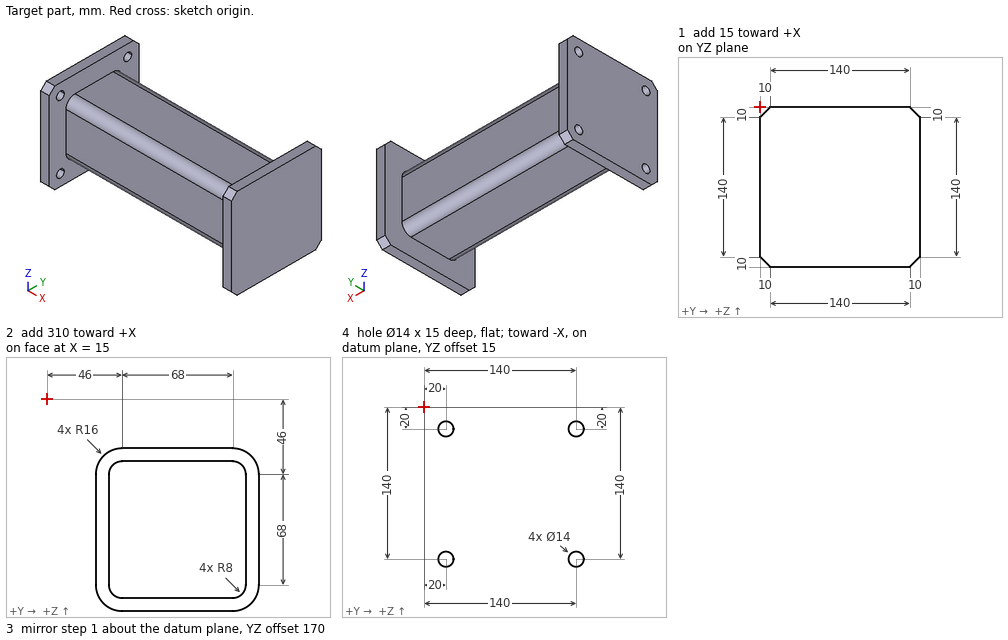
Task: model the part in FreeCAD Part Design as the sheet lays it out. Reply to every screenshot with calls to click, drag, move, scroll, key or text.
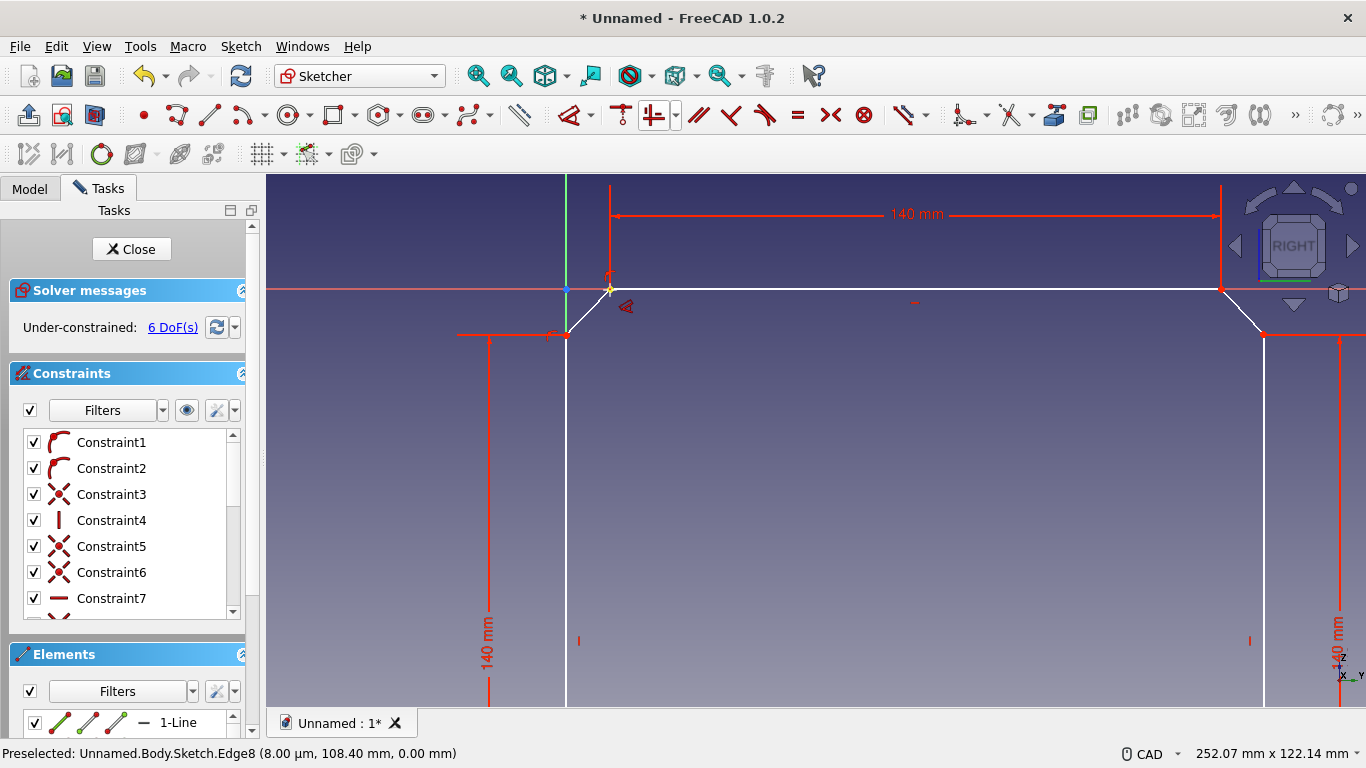
click(610, 289)
click(588, 255)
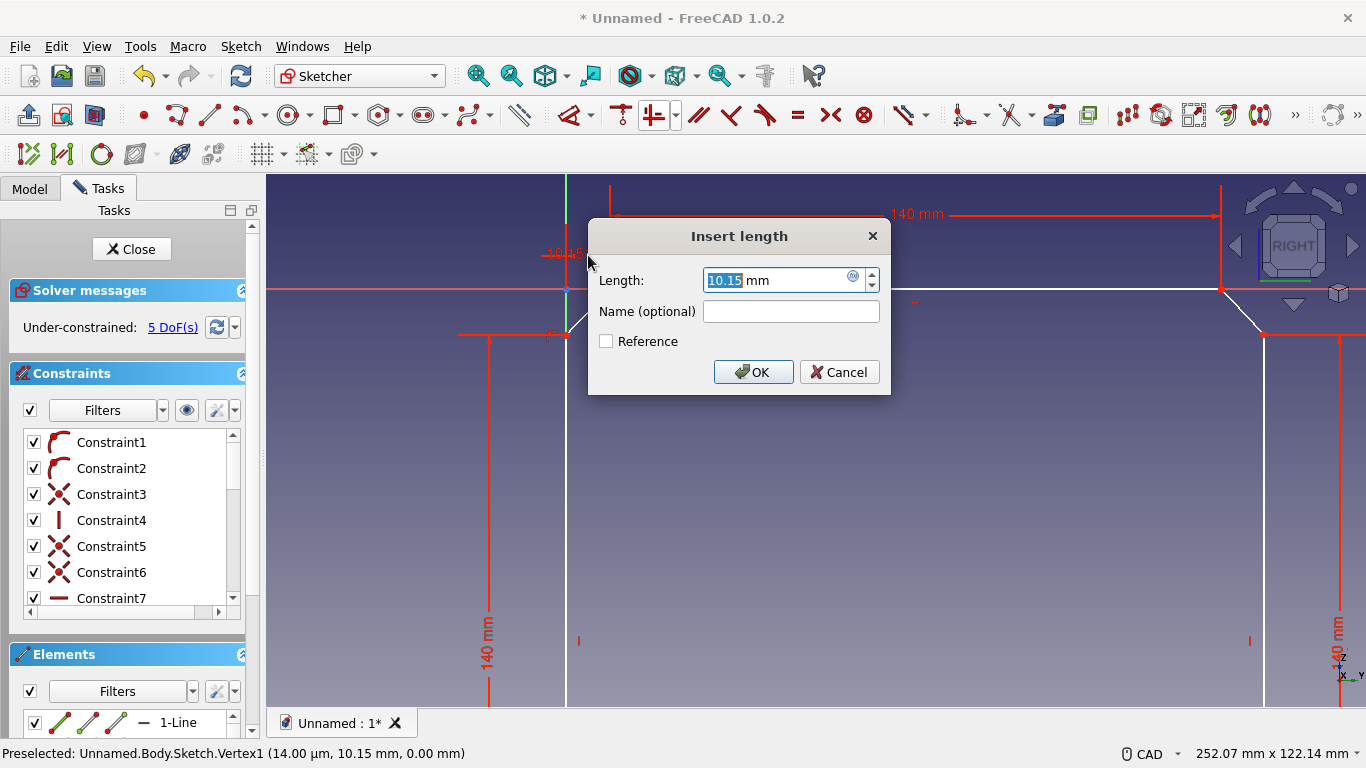
text(10)
key(Return)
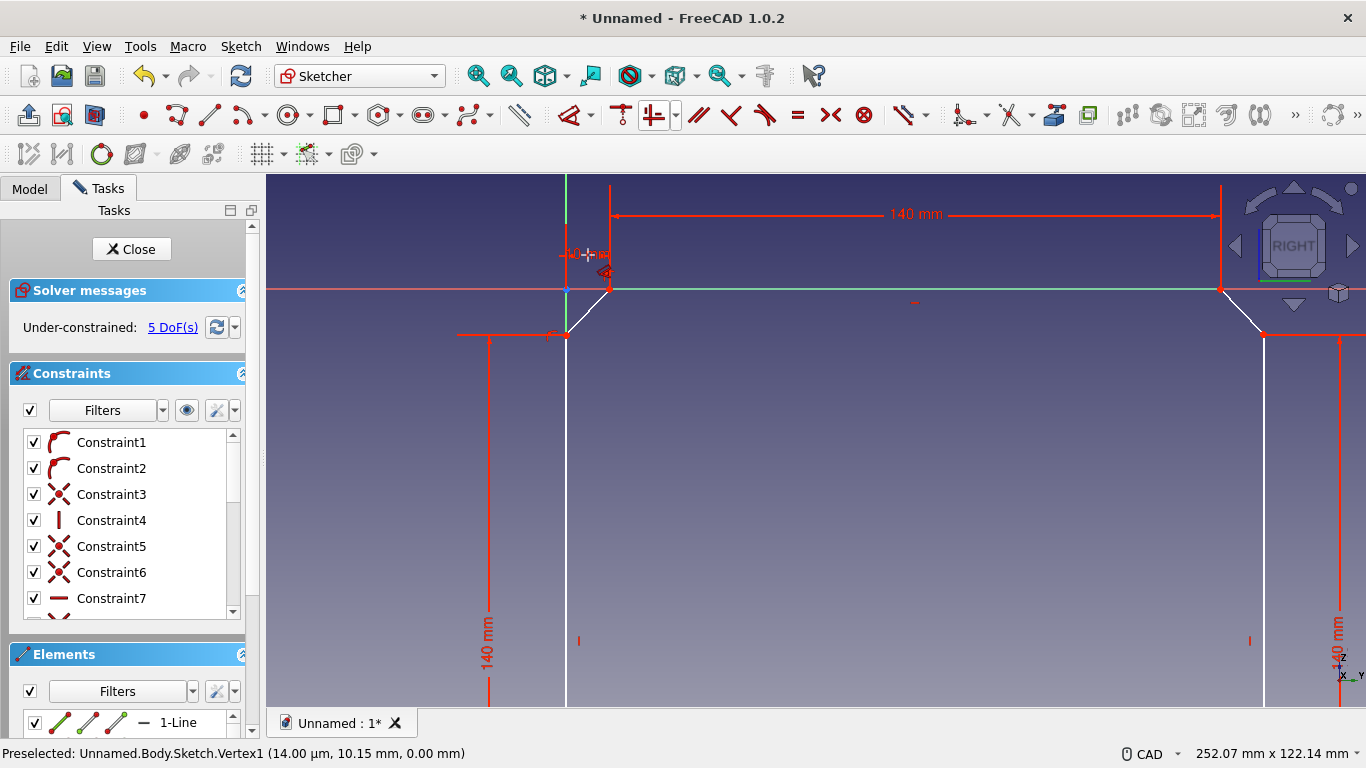
click(566, 335)
click(532, 312)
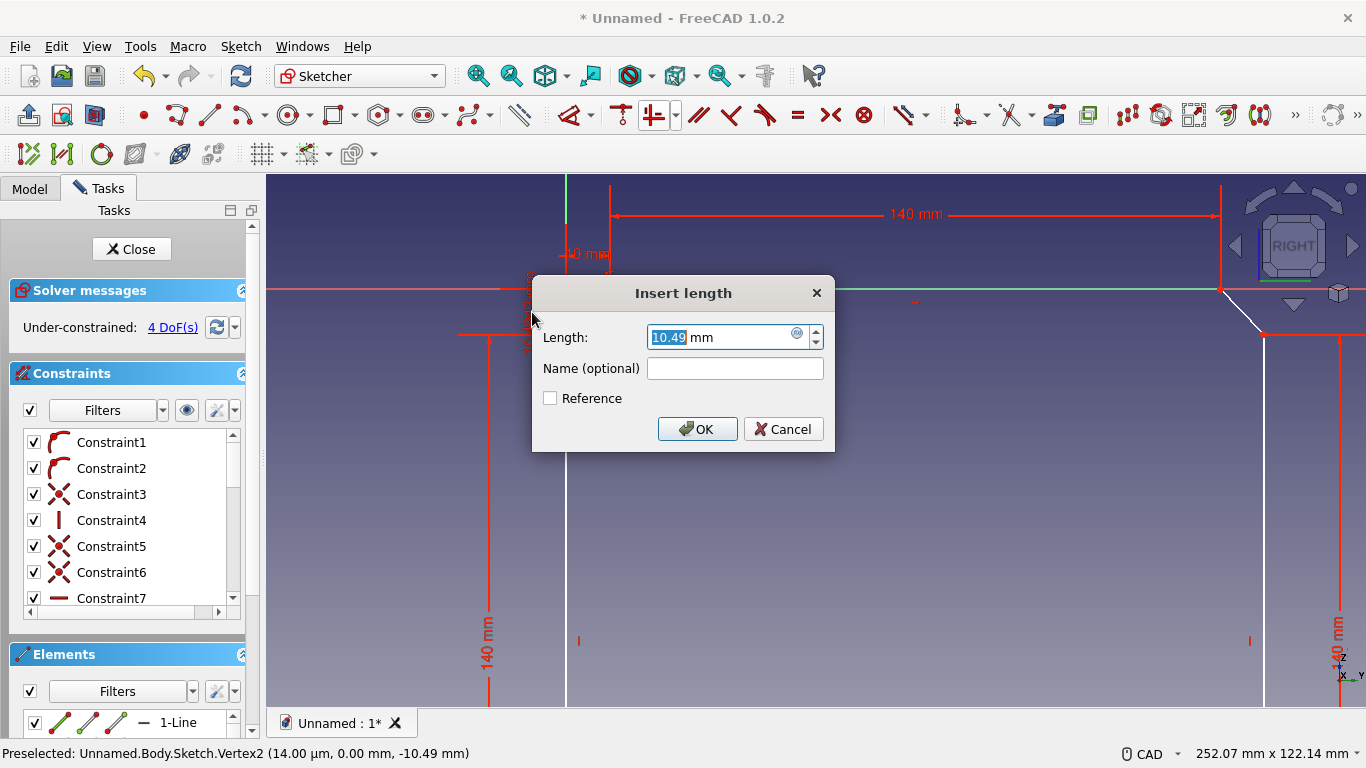
text(10)
key(Return)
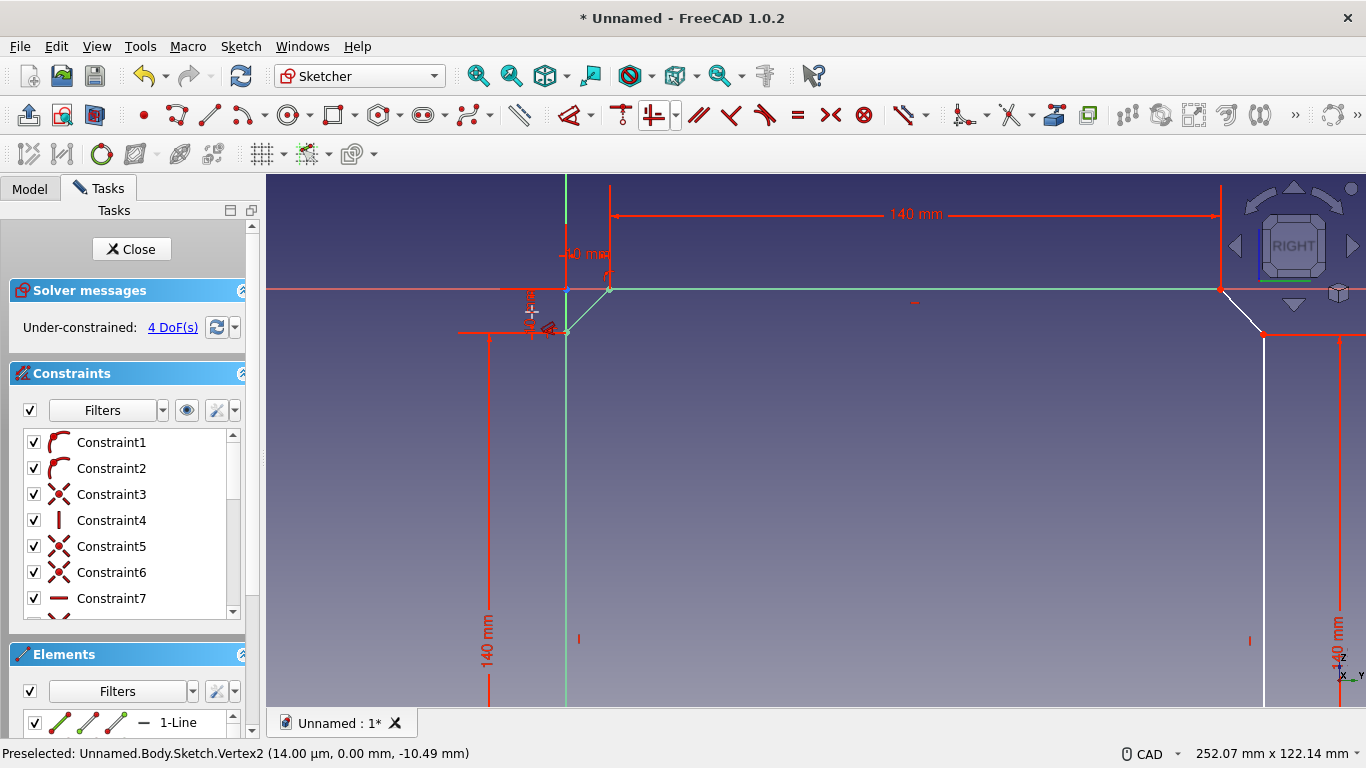
scroll(611, 279, down, 4)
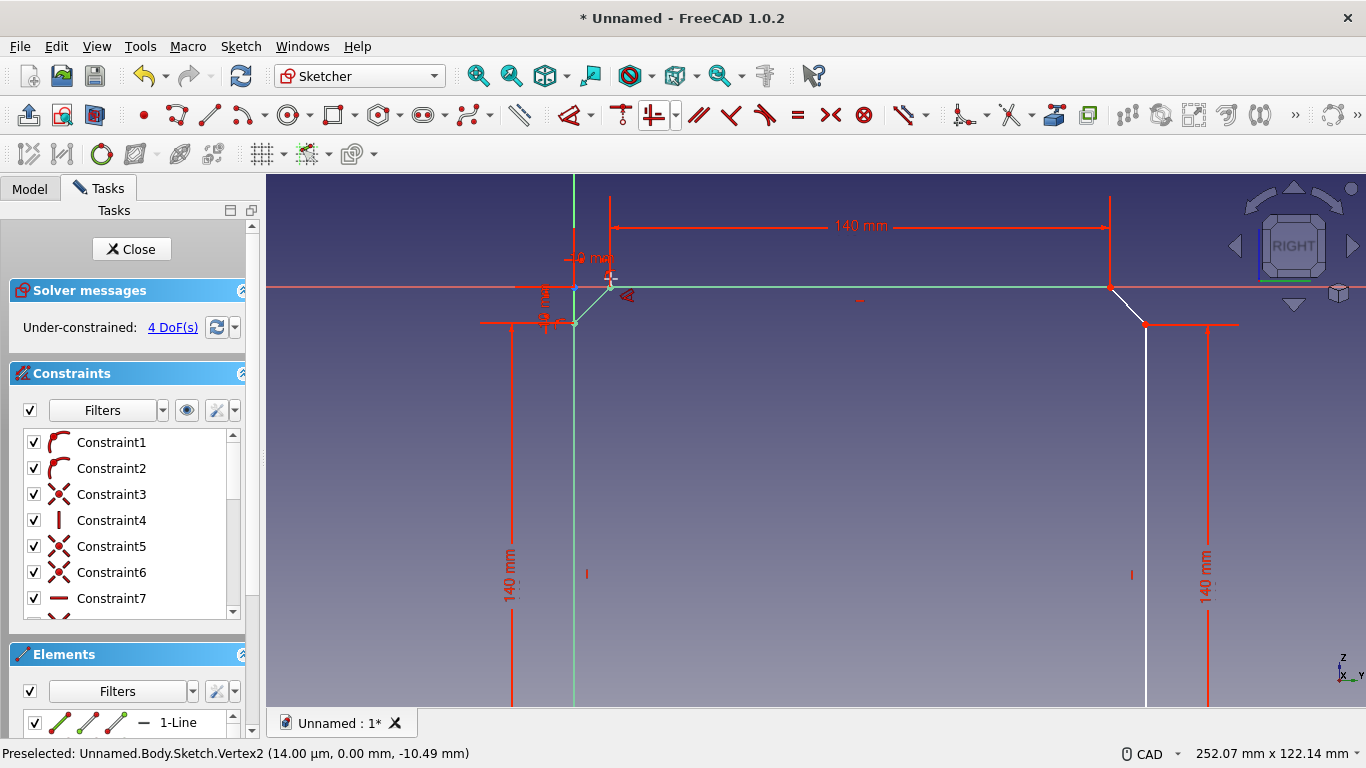
scroll(611, 599, up, 4)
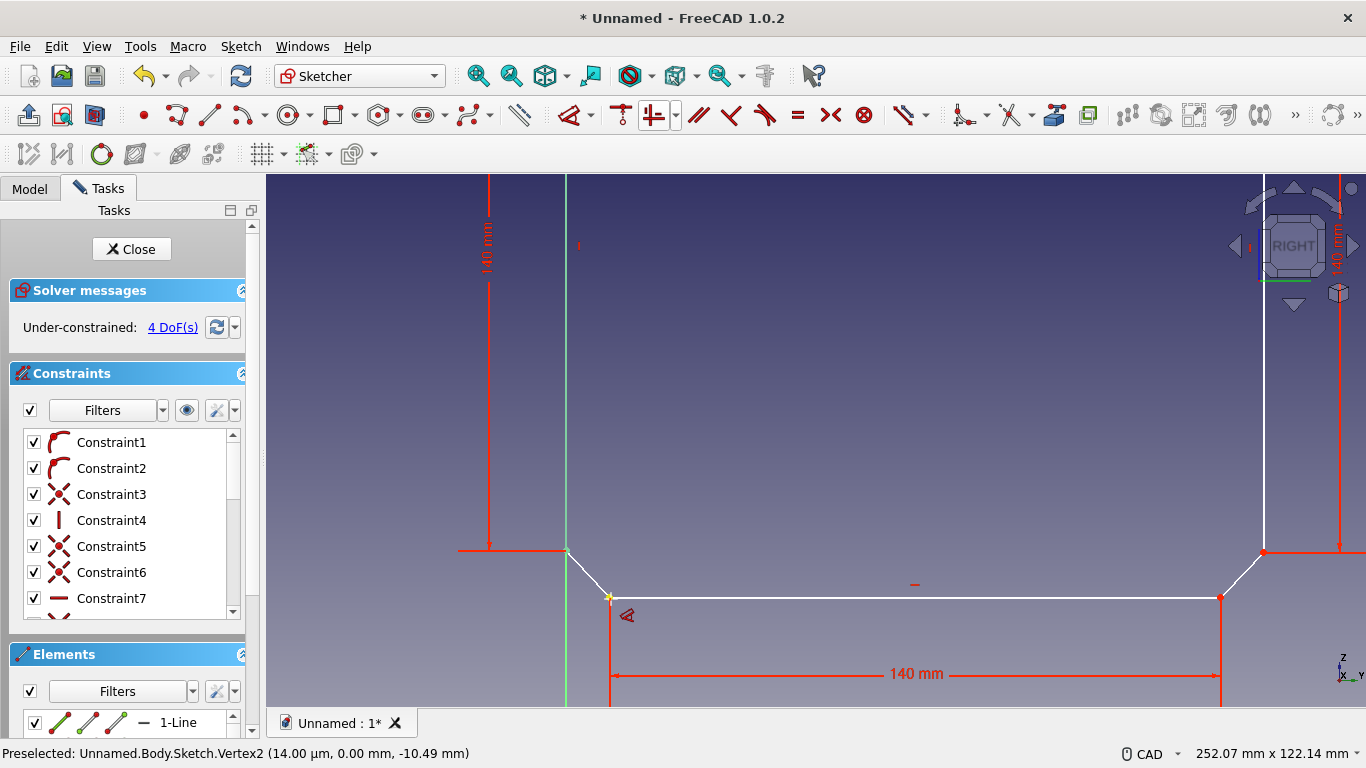
click(610, 598)
click(588, 632)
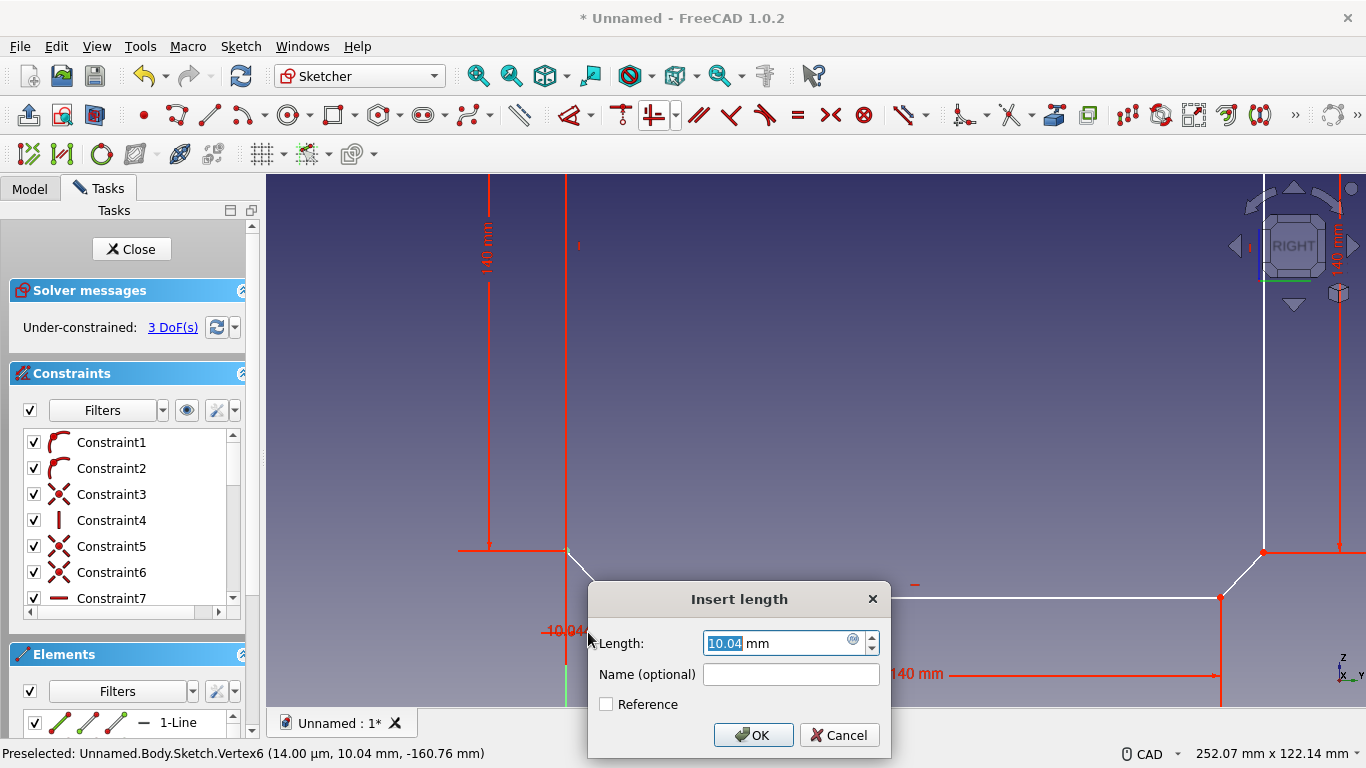
text(10)
key(Return)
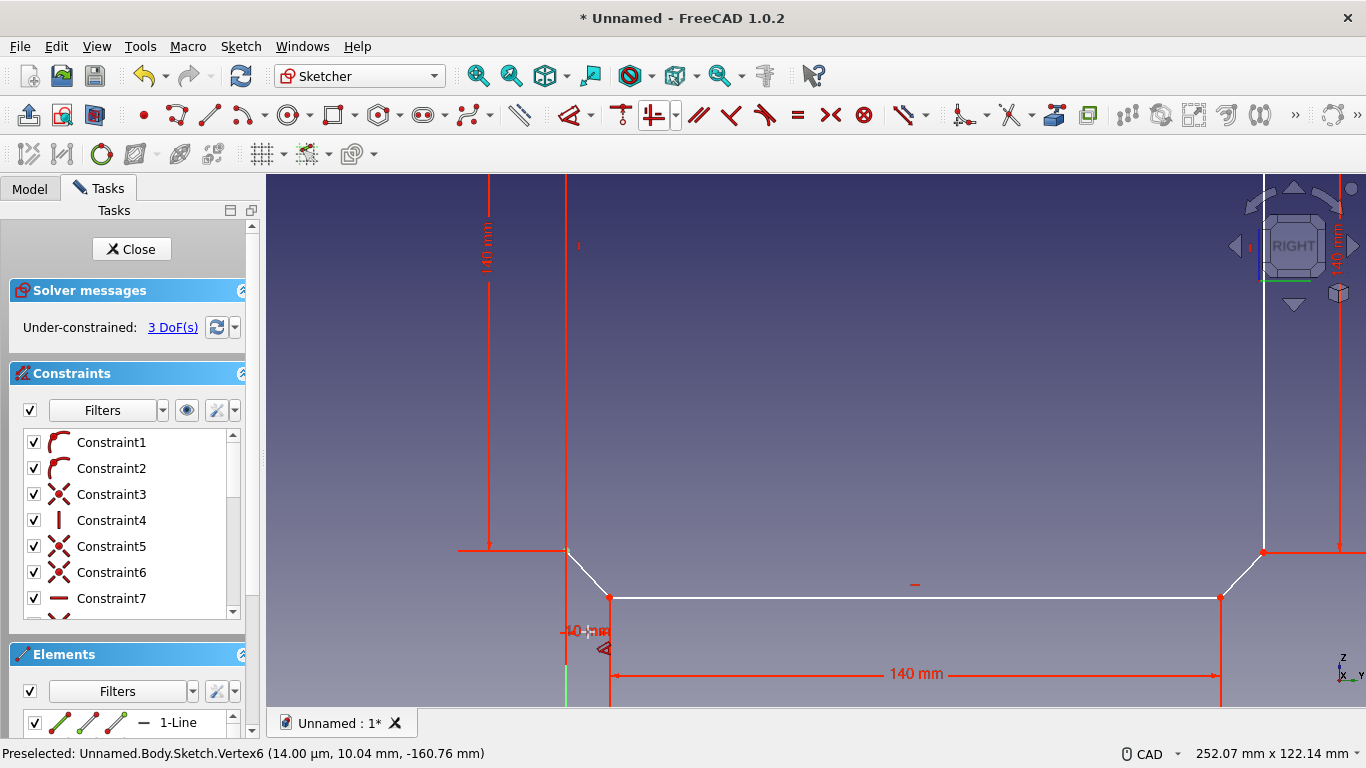
scroll(611, 600, down, 4)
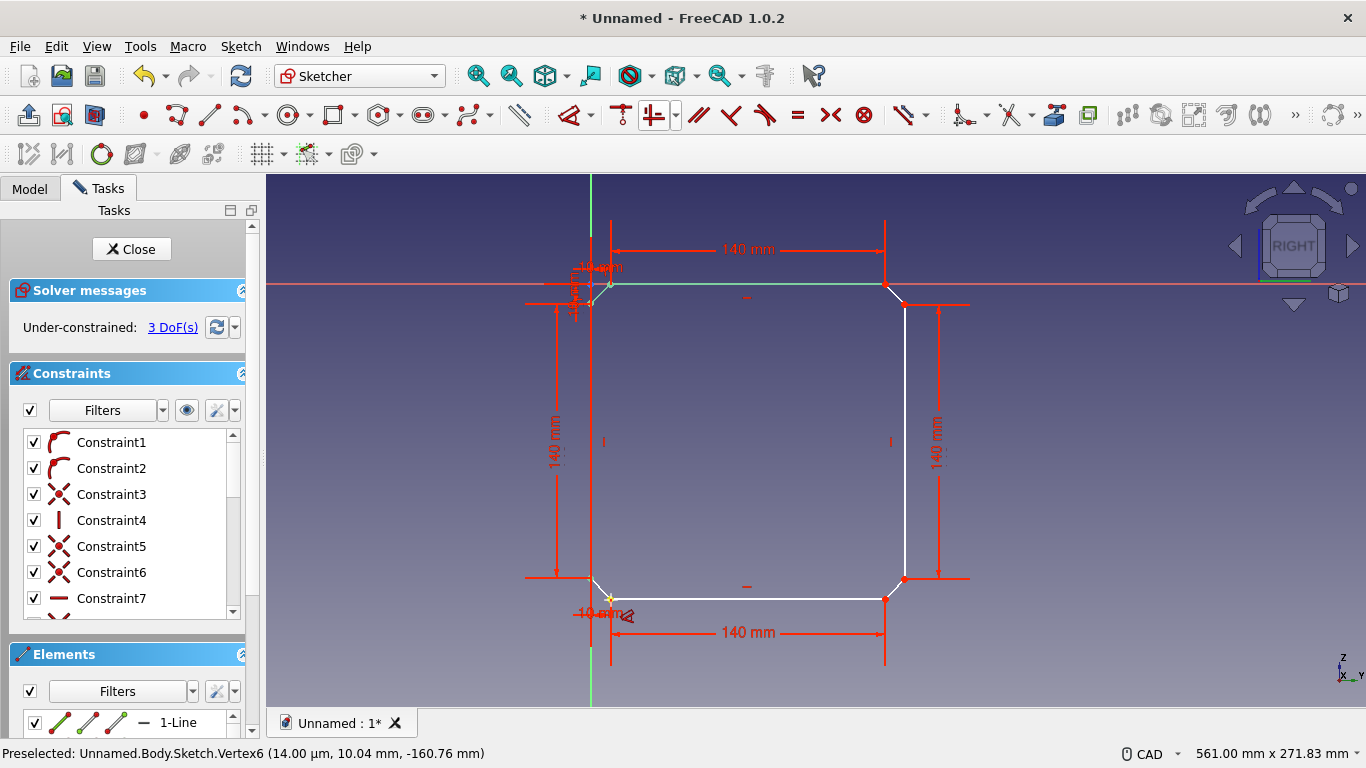
scroll(905, 305, up, 4)